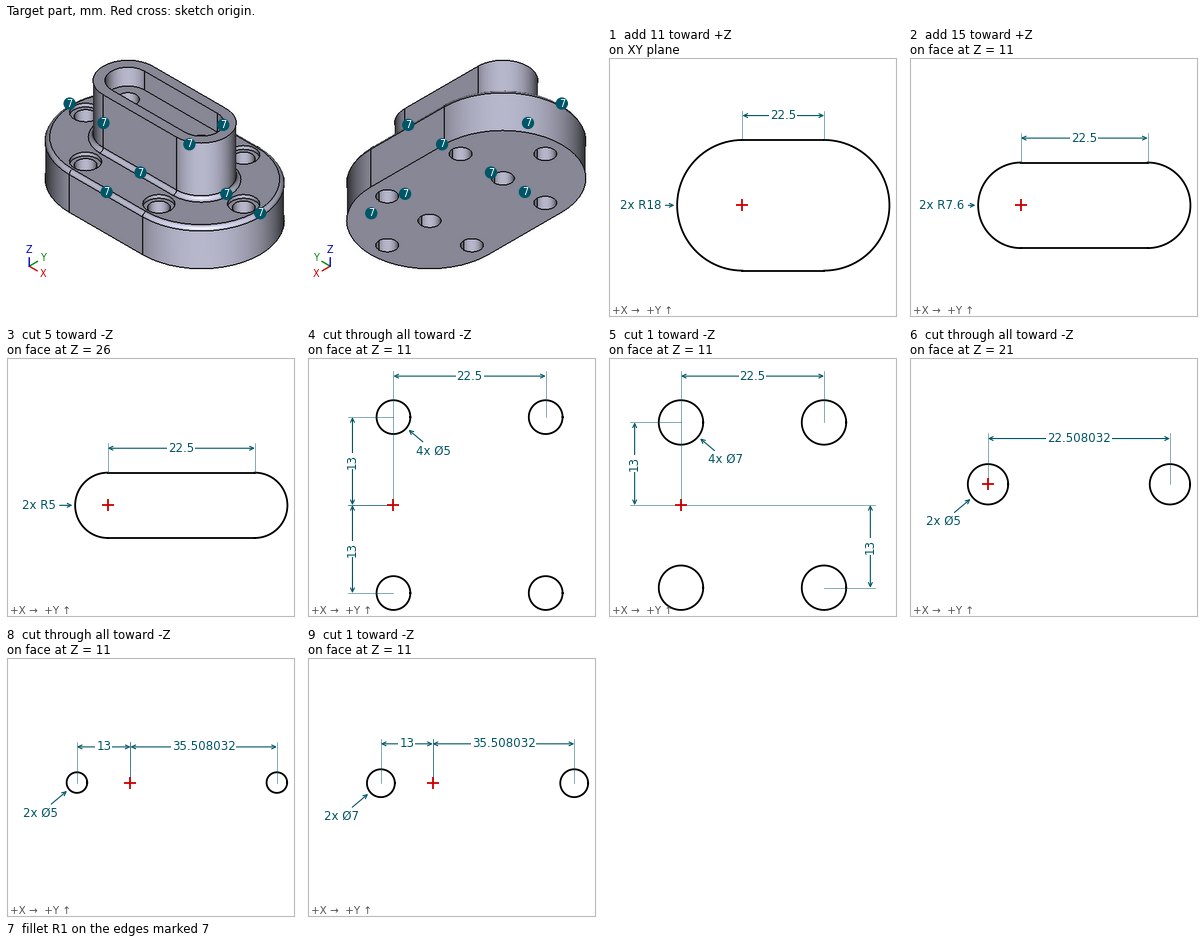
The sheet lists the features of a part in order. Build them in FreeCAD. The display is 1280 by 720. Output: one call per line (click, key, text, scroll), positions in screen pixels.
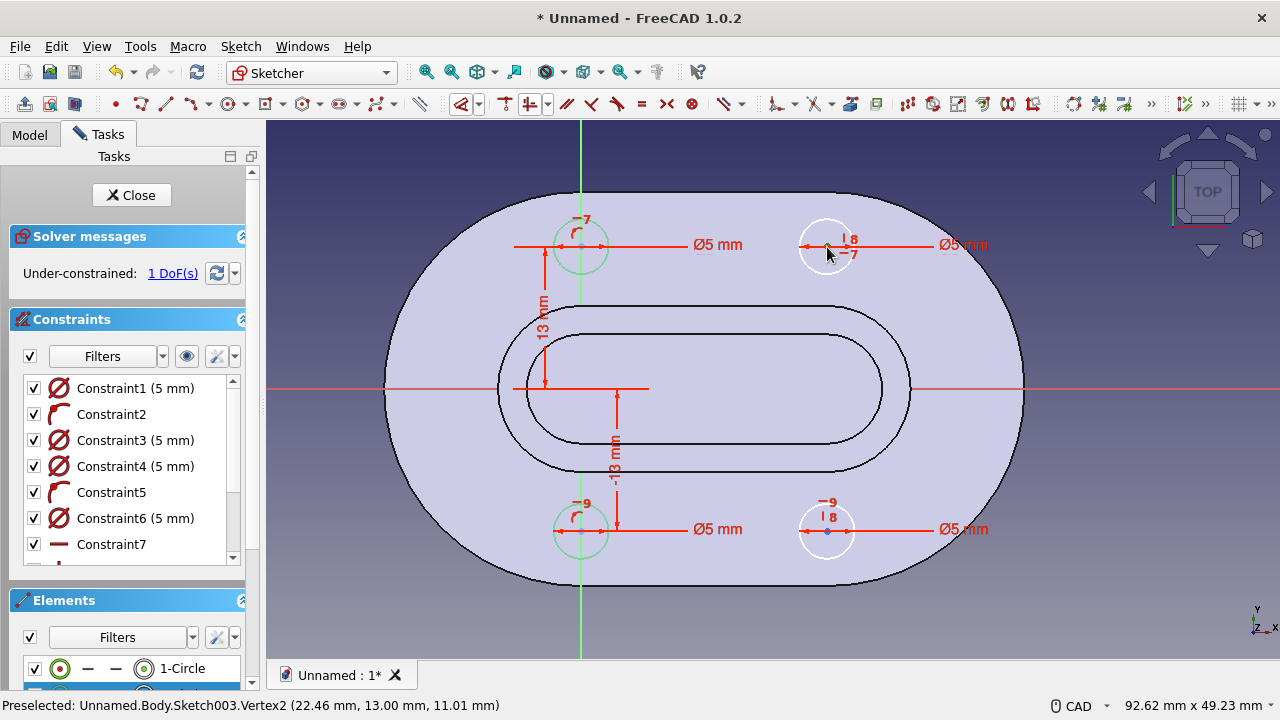
click(478, 104)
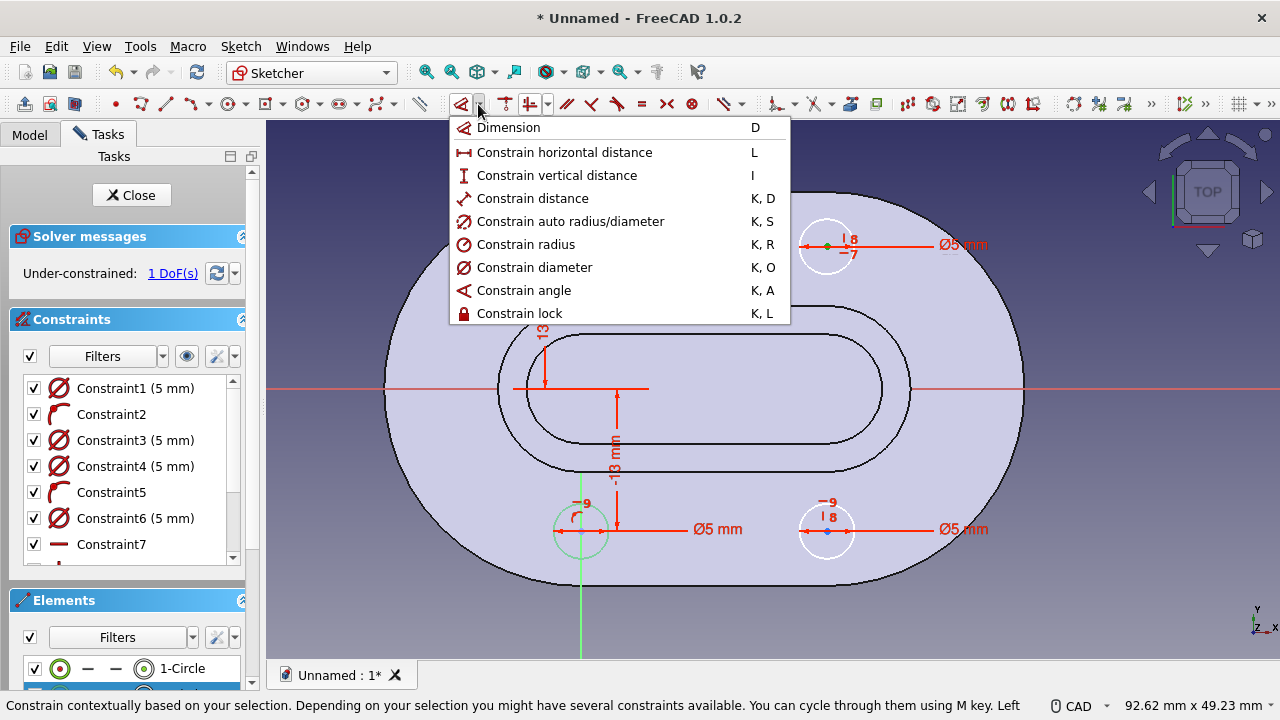
click(620, 152)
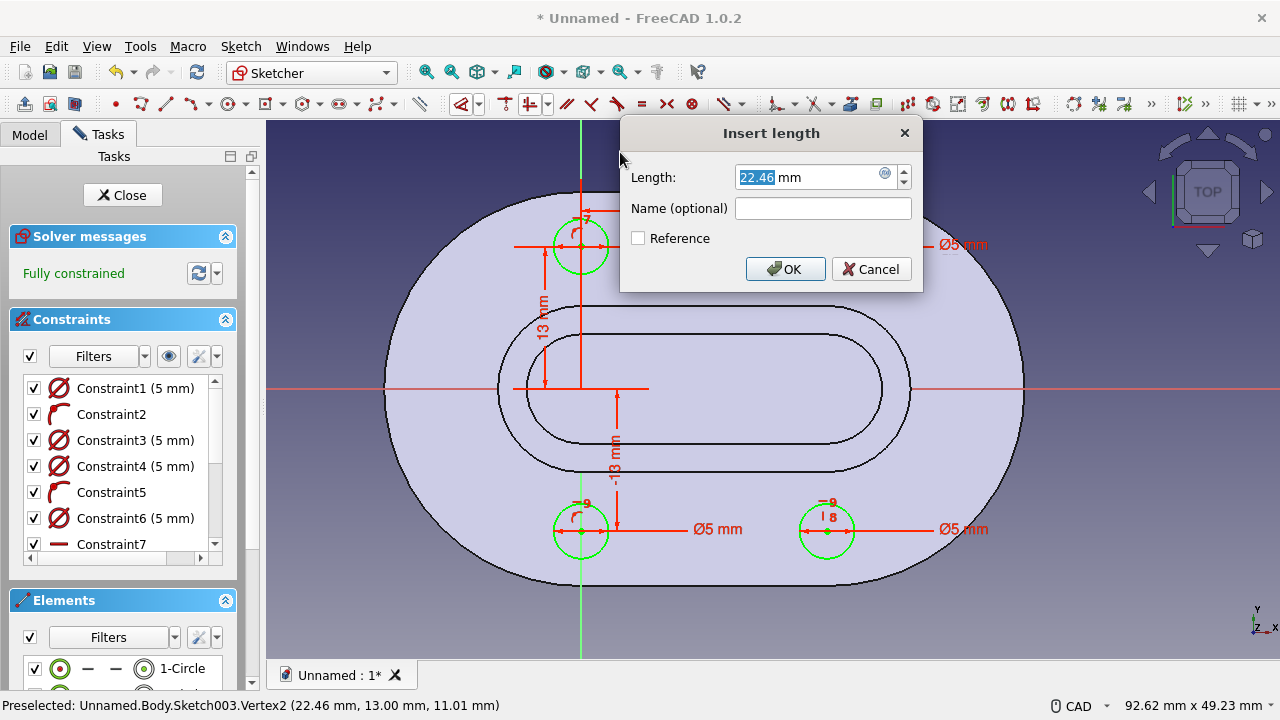
text(22.5)
key(Return)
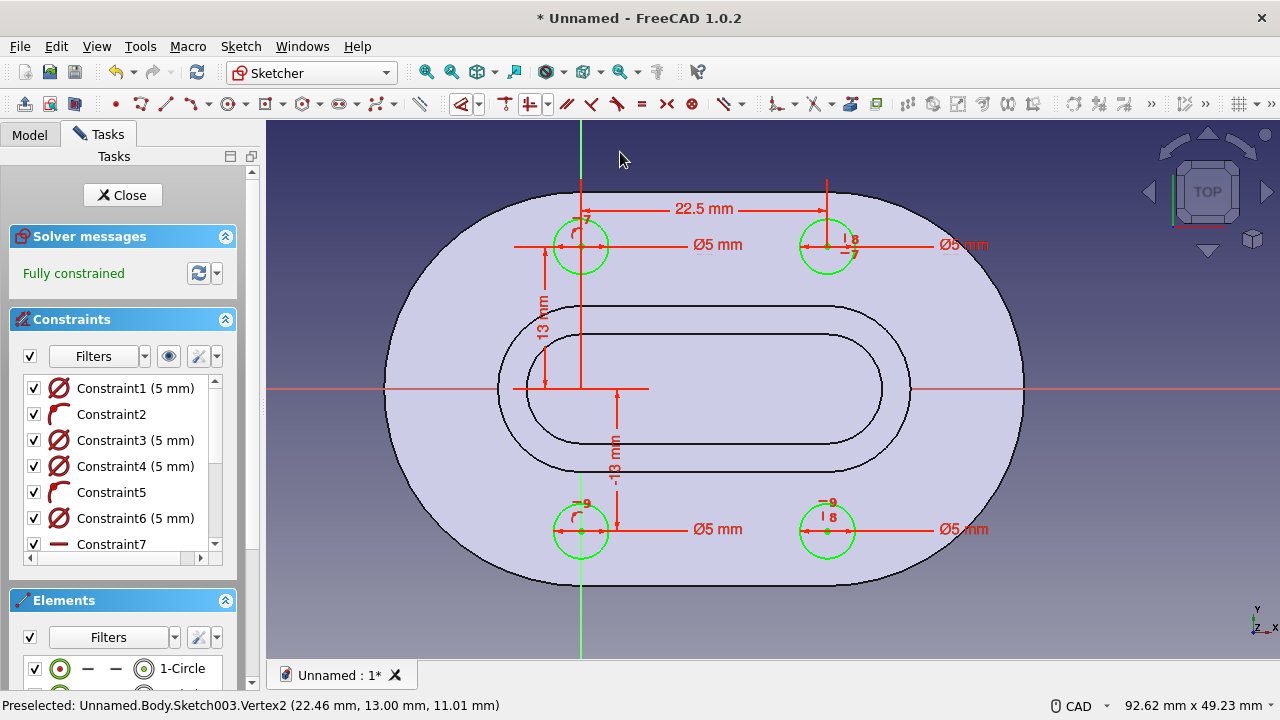
click(123, 195)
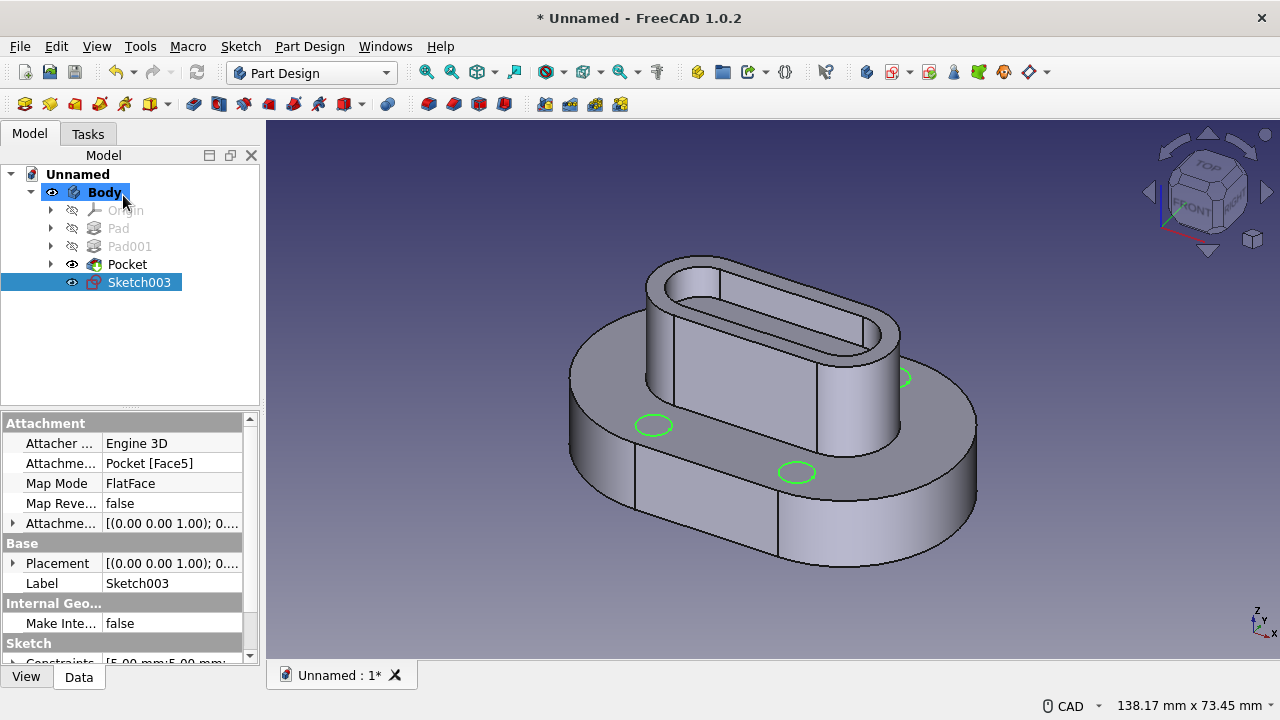
click(194, 104)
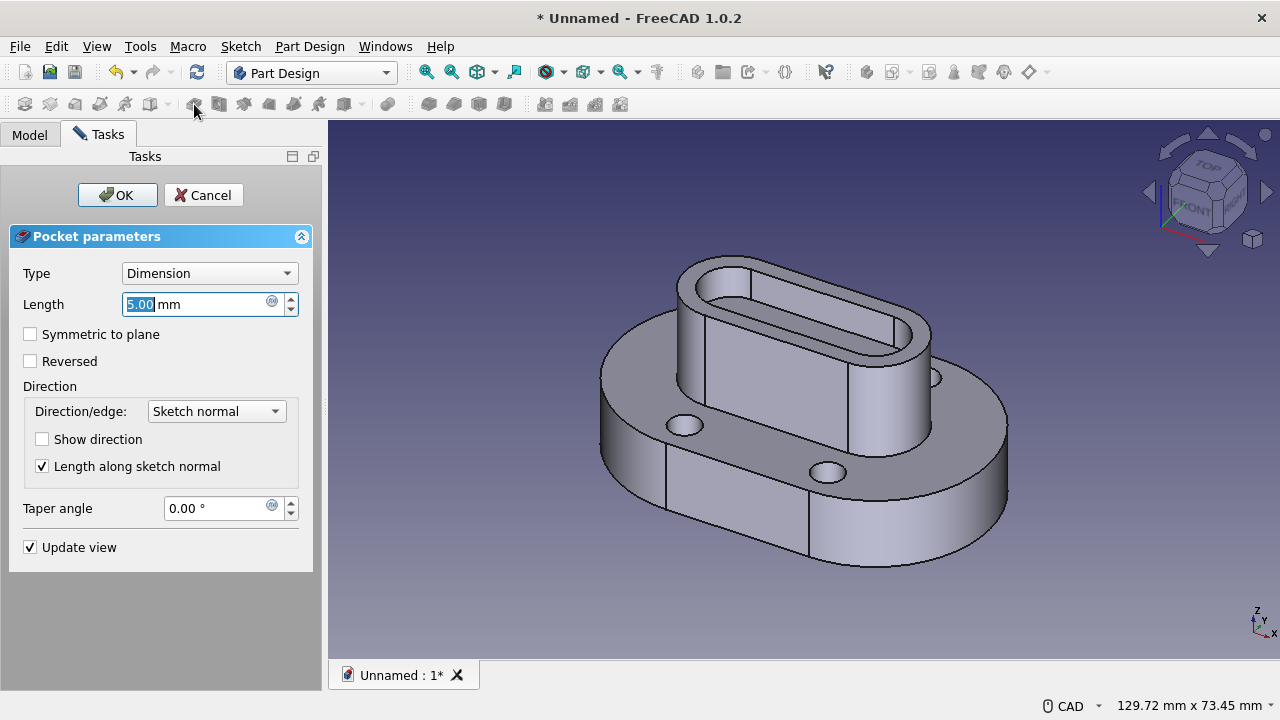
click(210, 274)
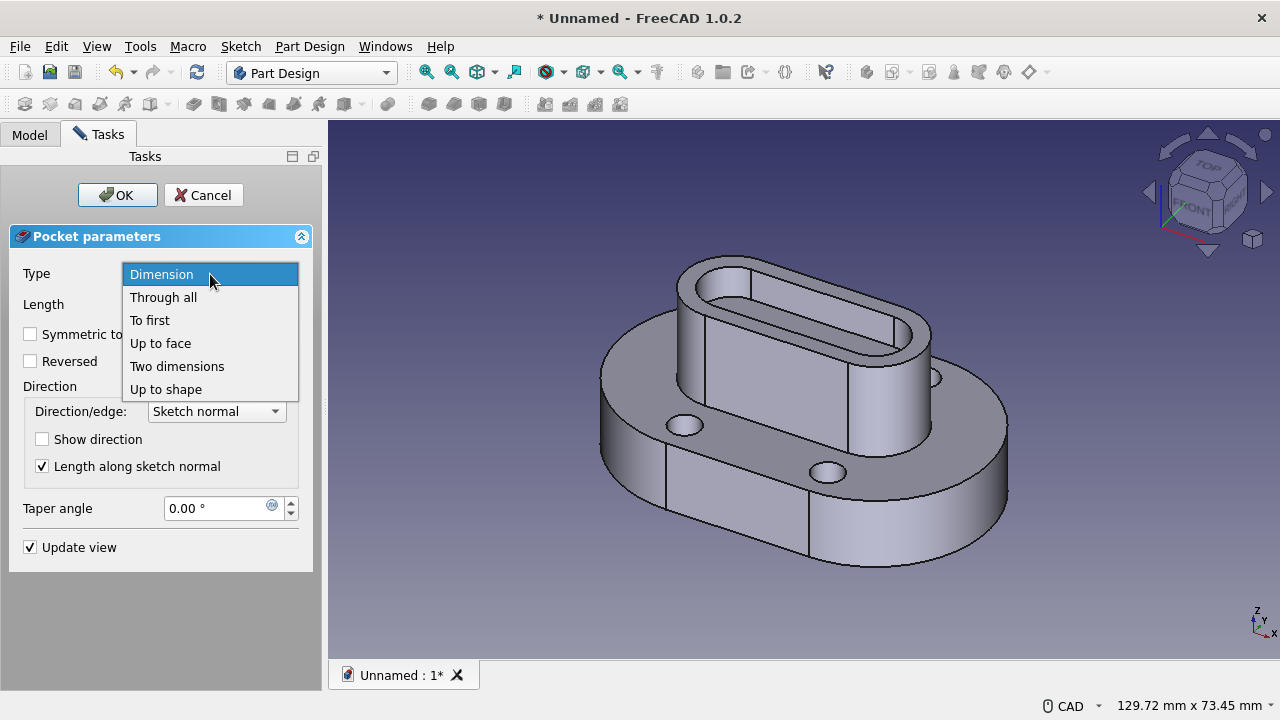
click(208, 298)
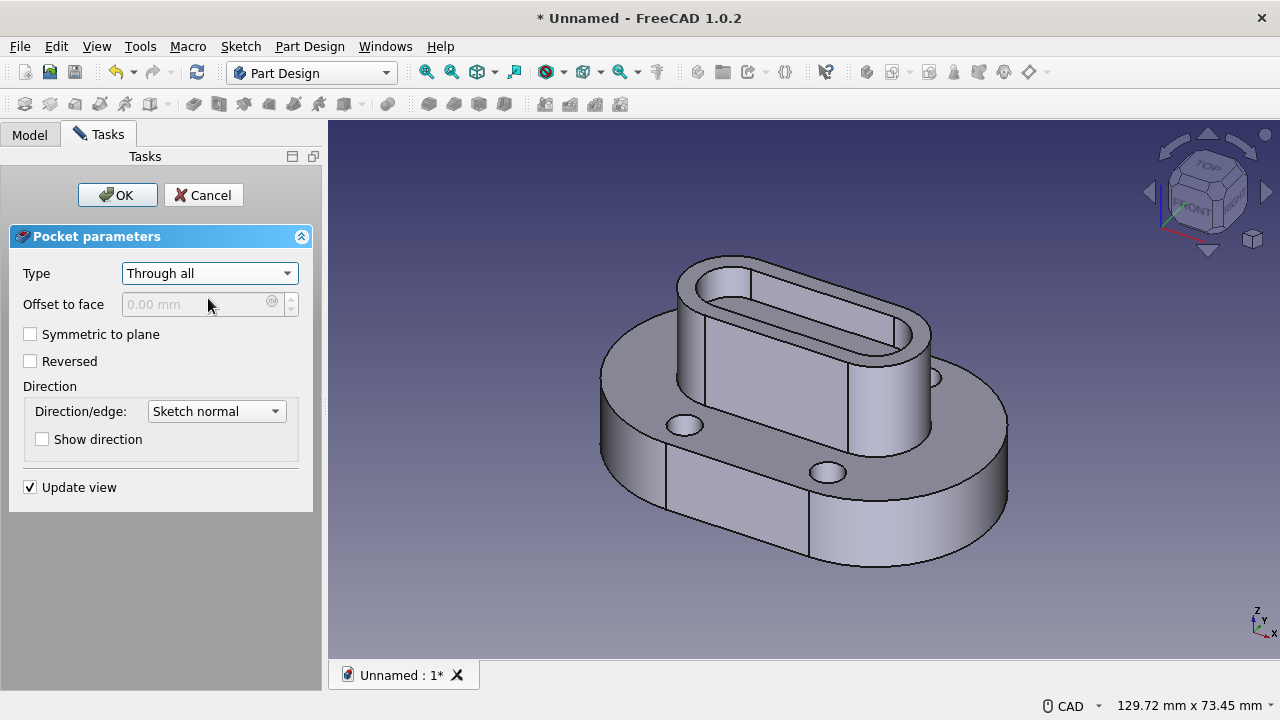
click(118, 195)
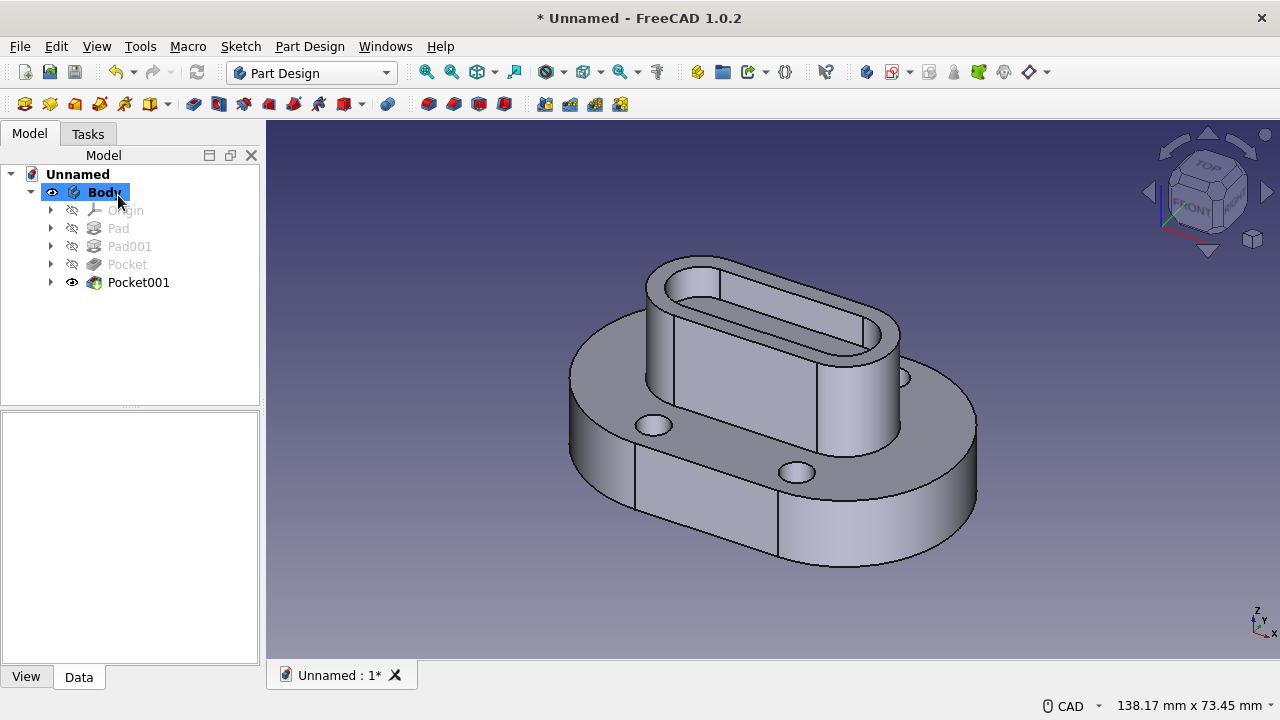
click(932, 453)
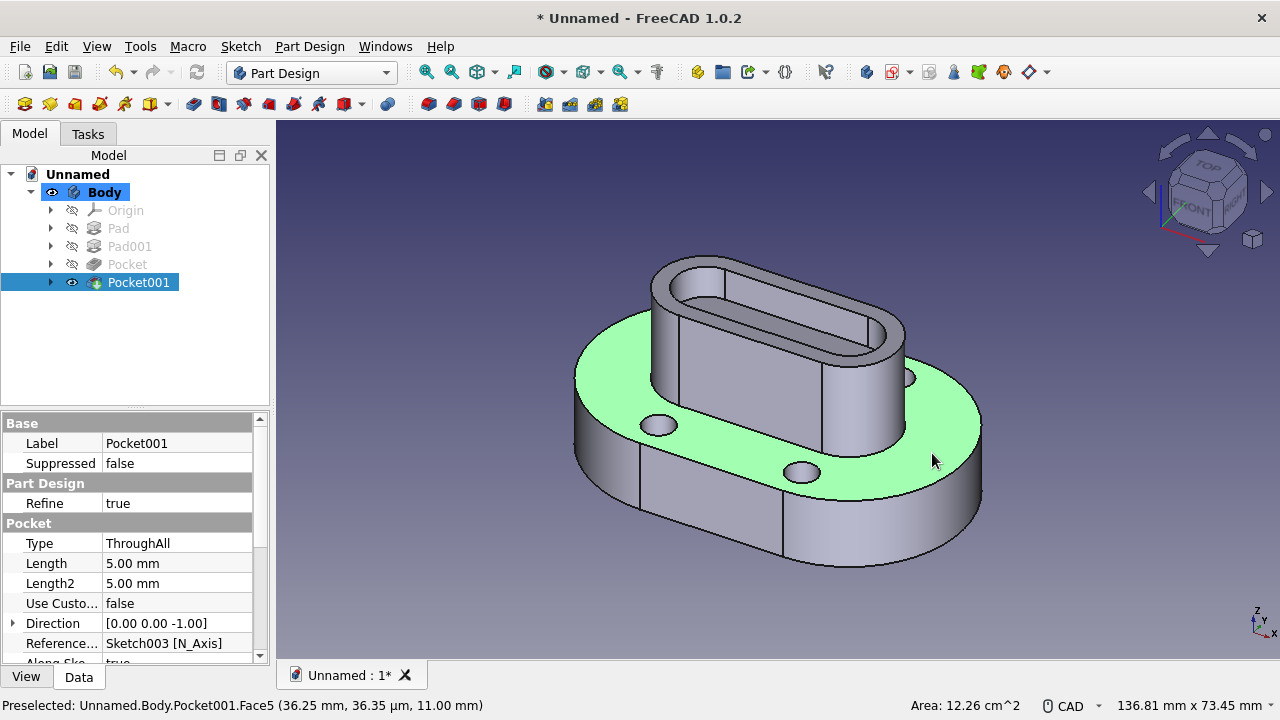
click(892, 72)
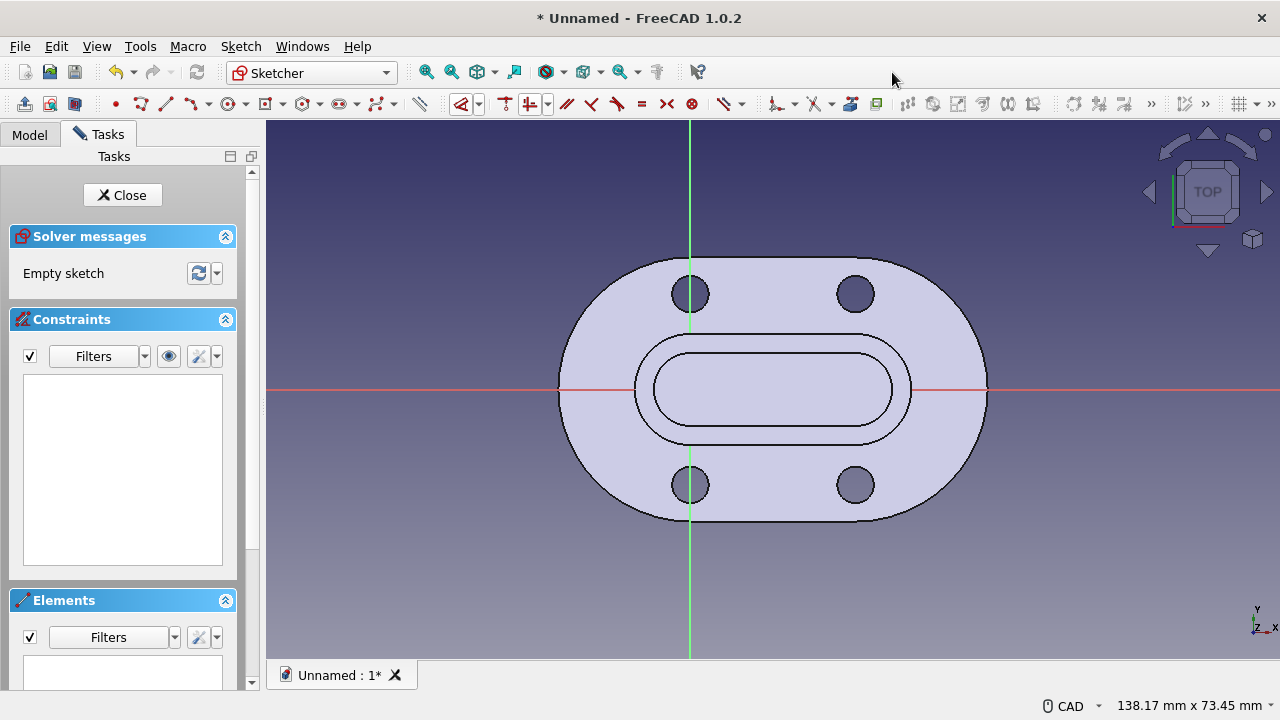
click(75, 104)